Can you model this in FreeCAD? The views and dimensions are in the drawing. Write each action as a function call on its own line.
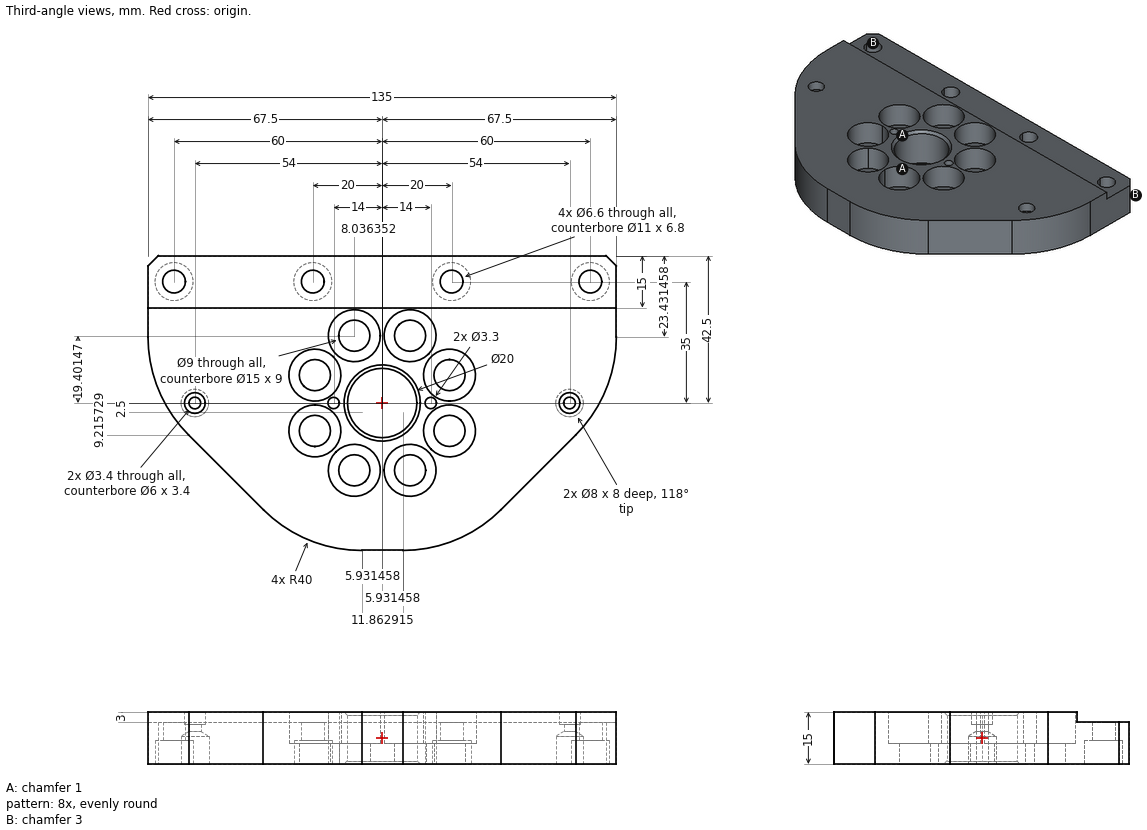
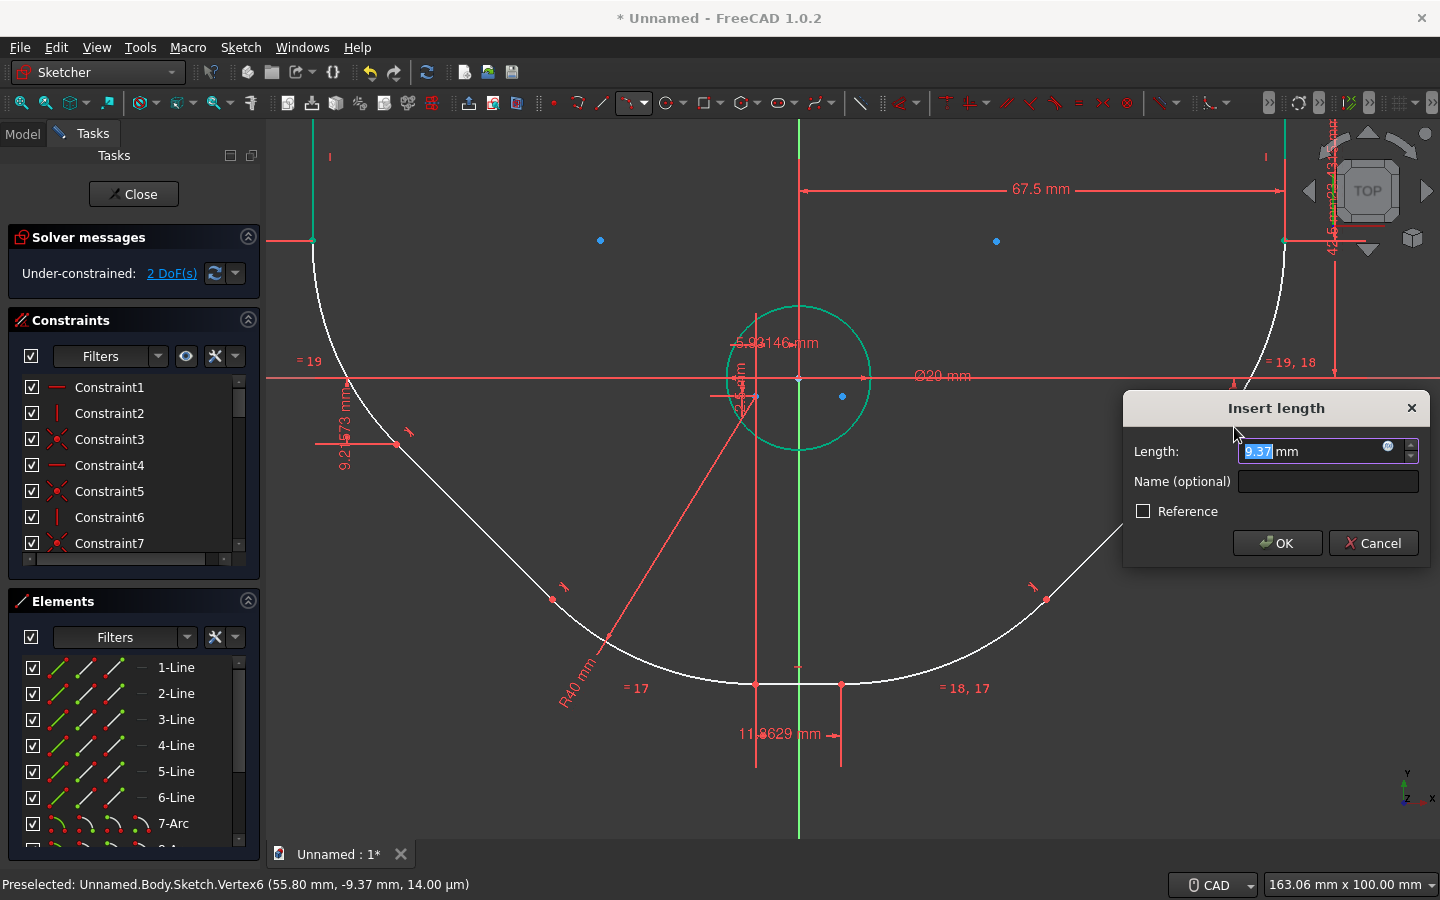
text(9.215729)
key(Return)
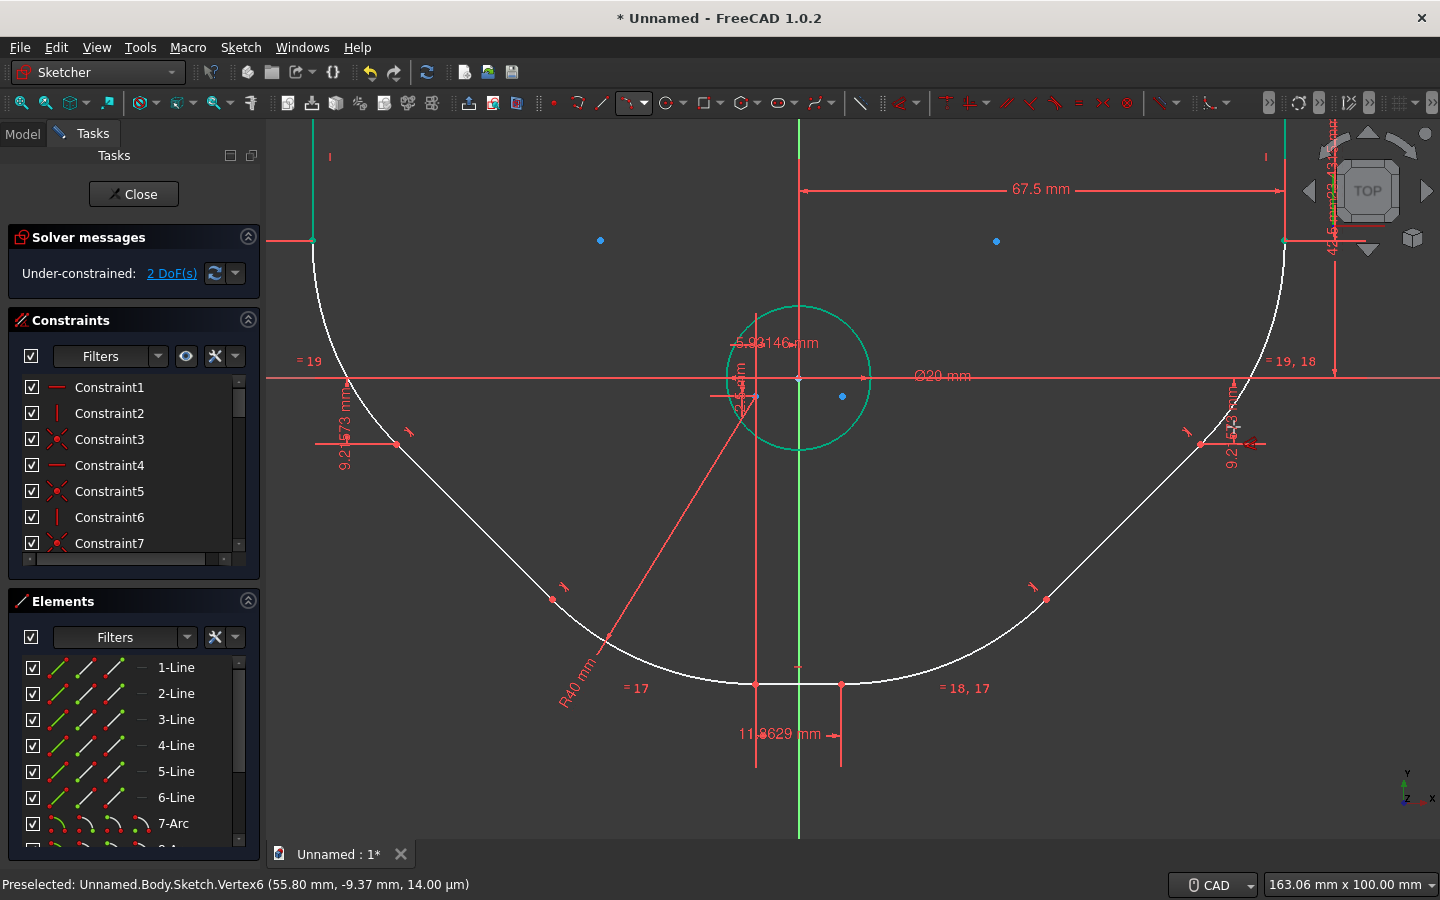
click(756, 396)
click(777, 430)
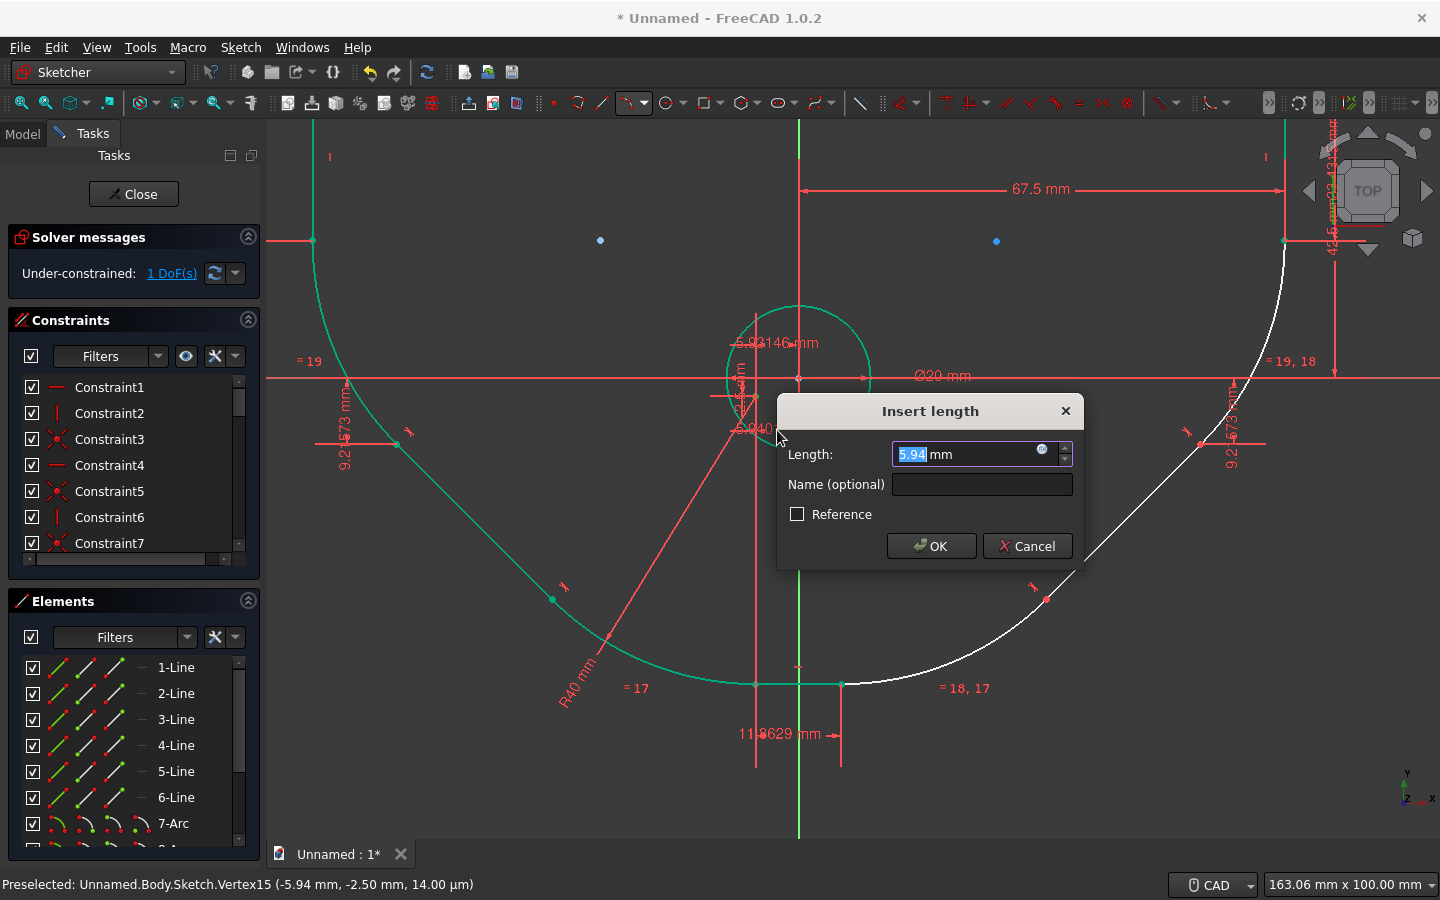
text(5.931458)
key(Return)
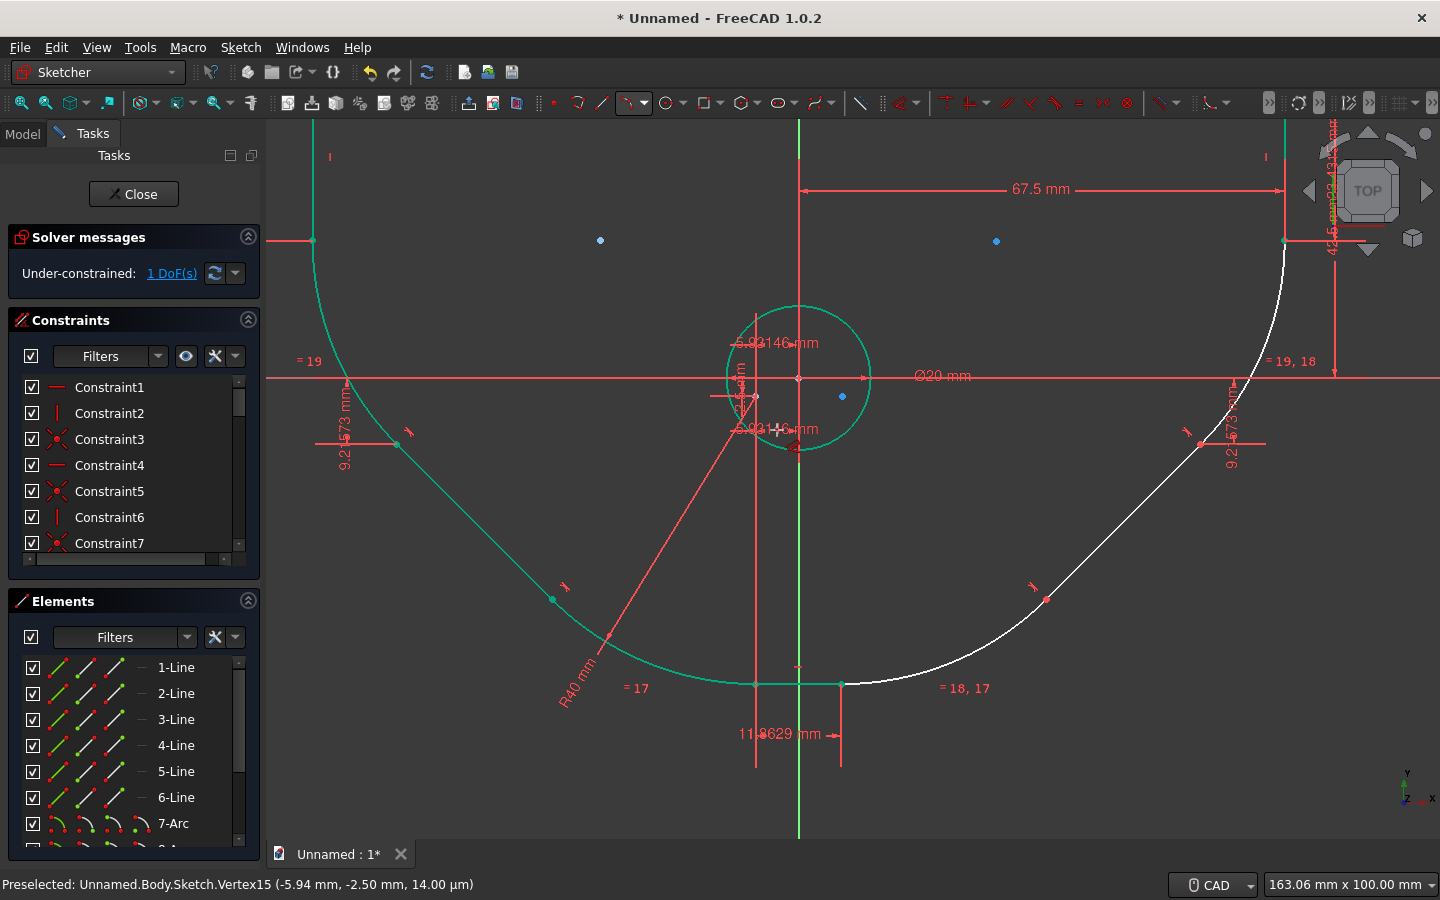
click(842, 396)
click(821, 478)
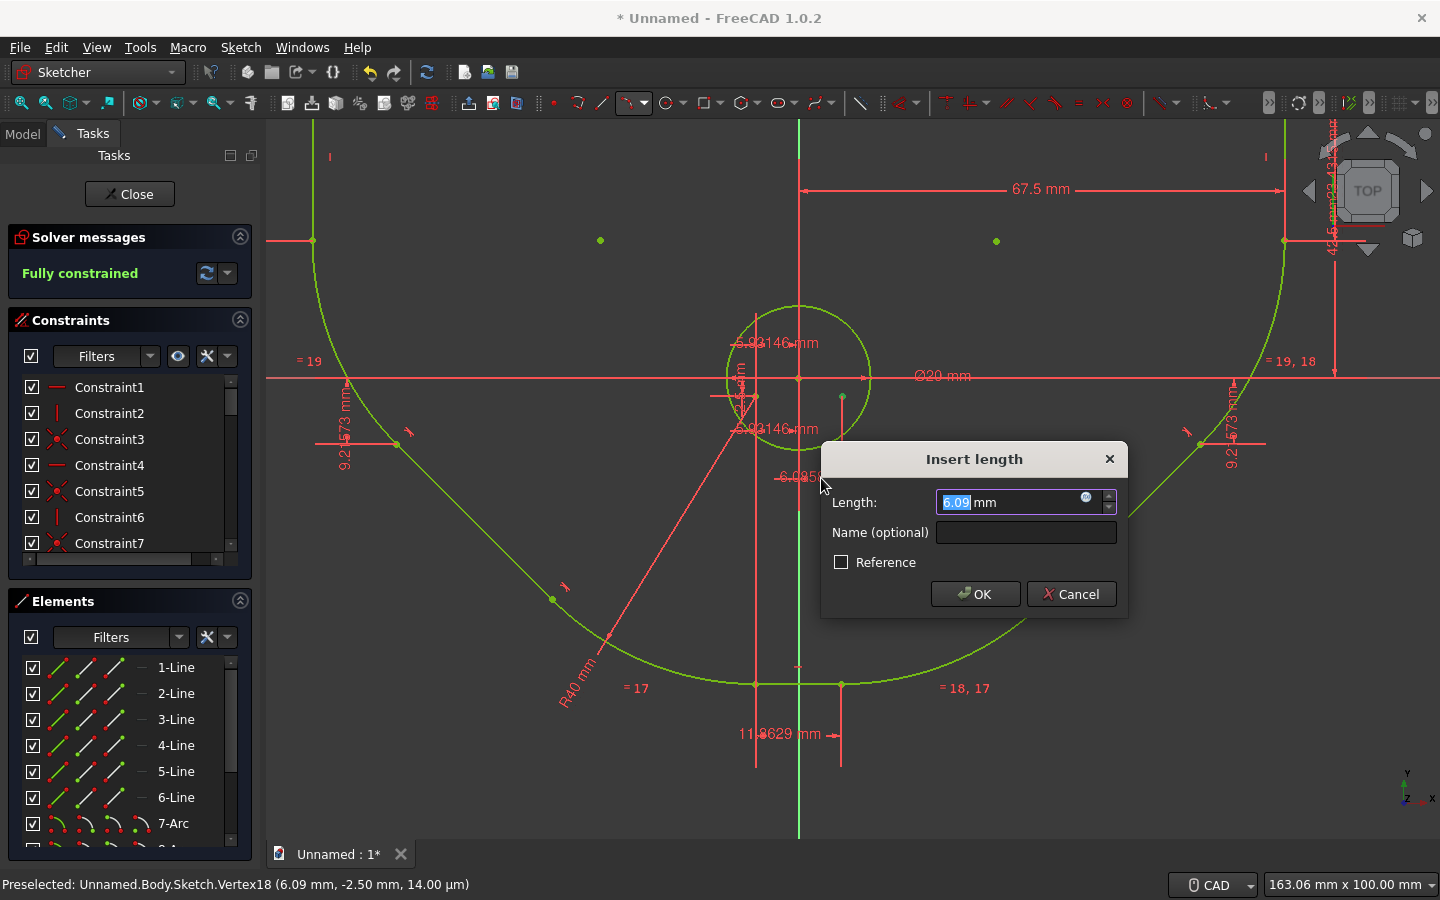
text(5.931458)
key(Return)
key(Escape)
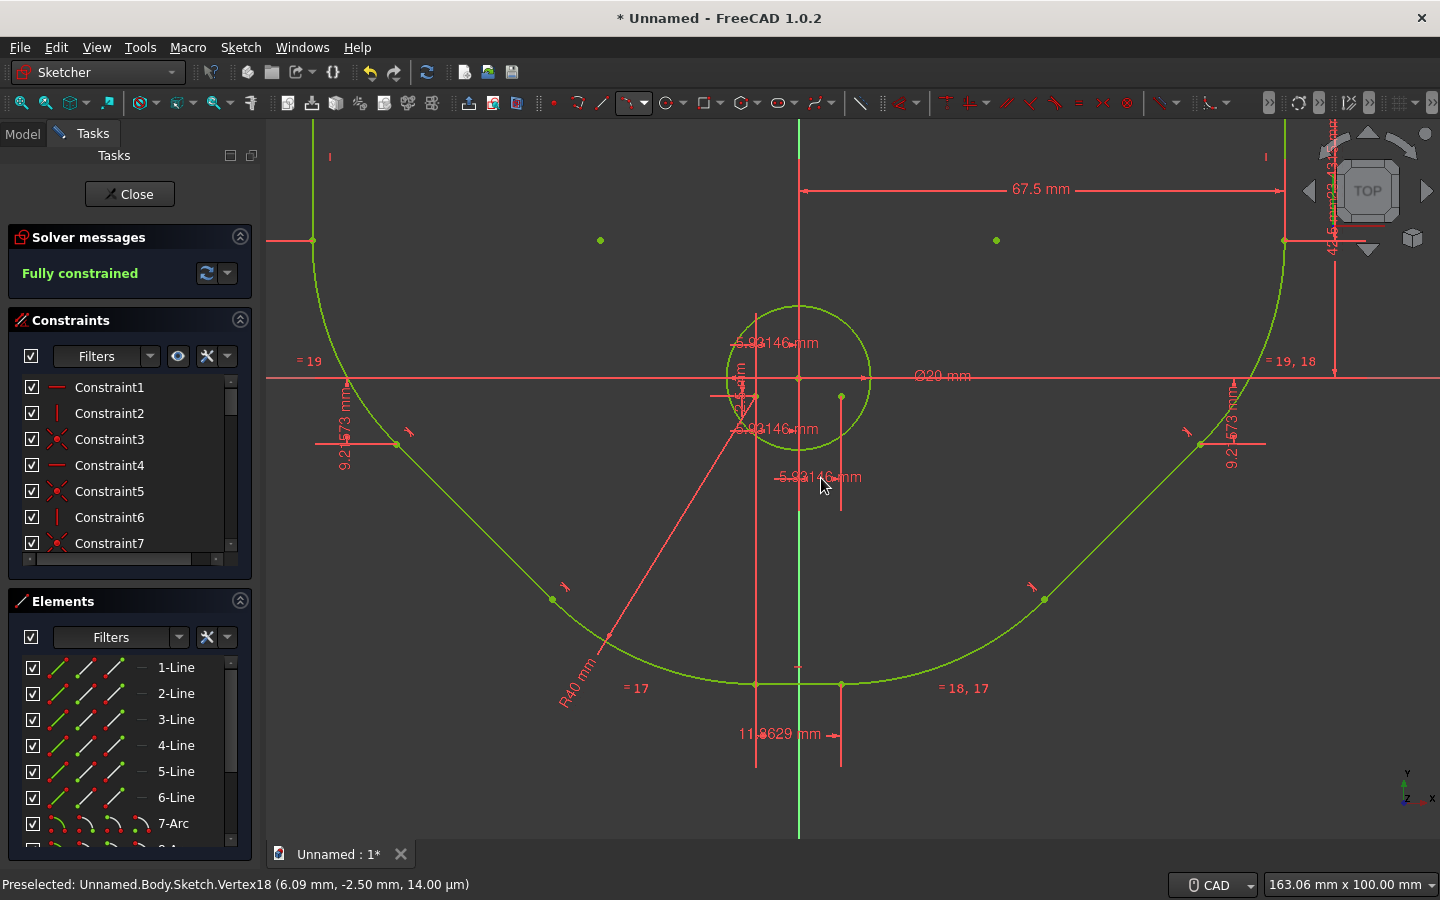
click(130, 194)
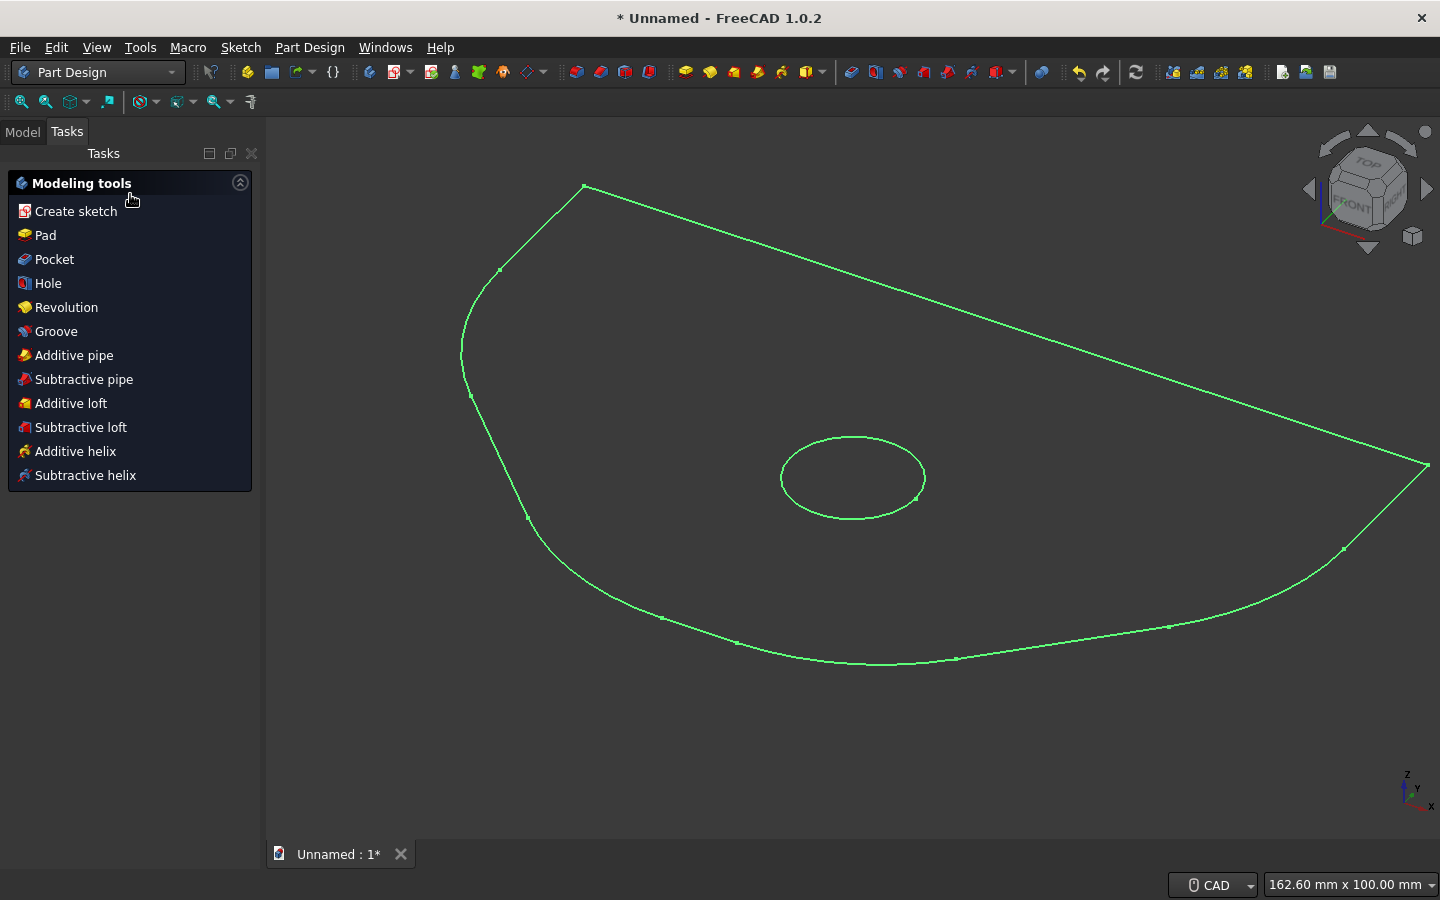
click(686, 72)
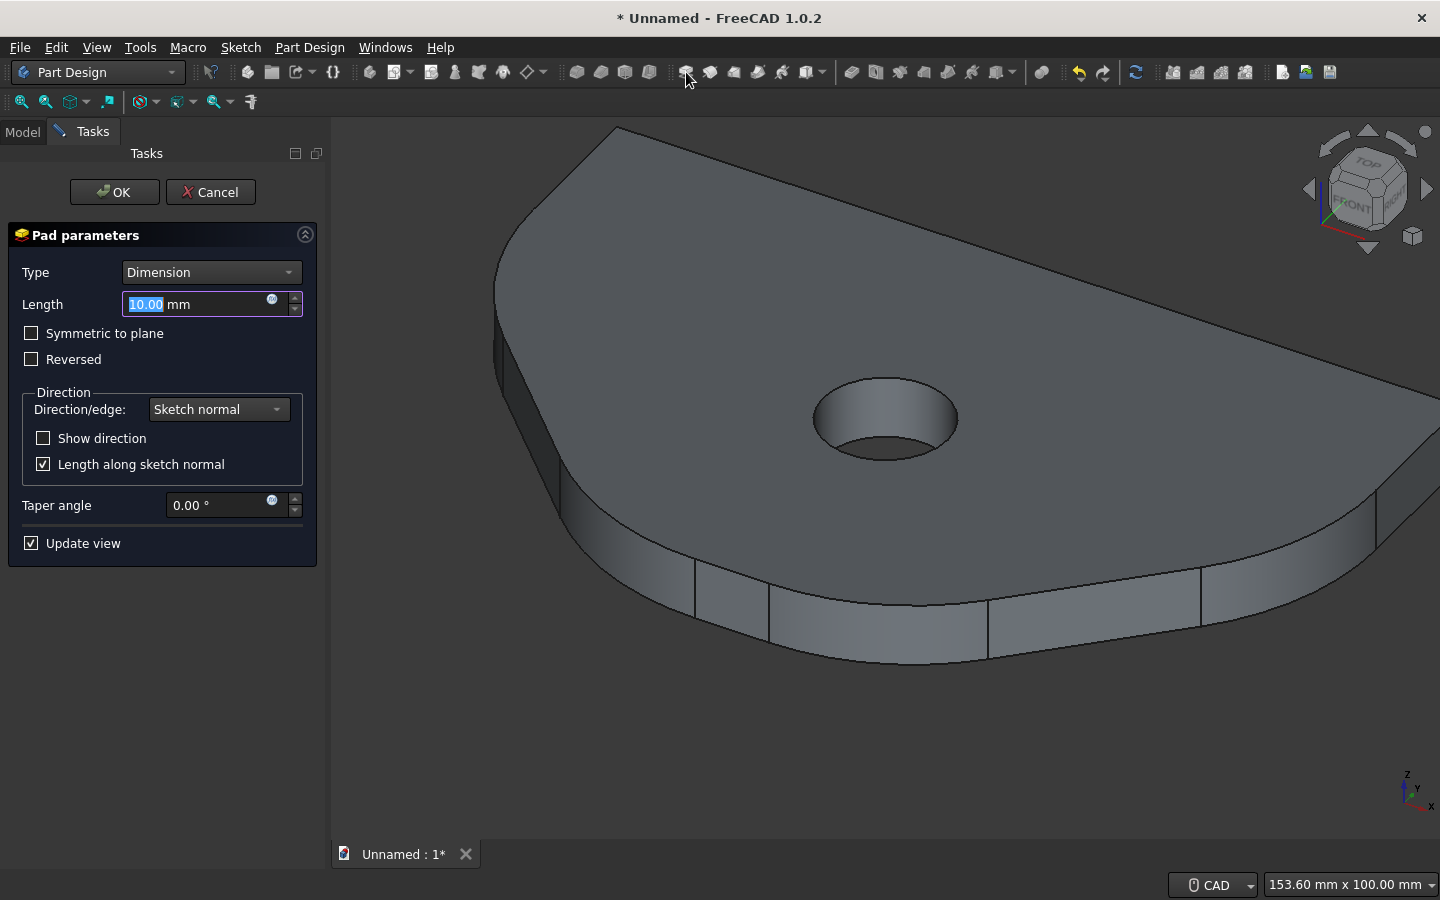
text(15)
key(Tab)